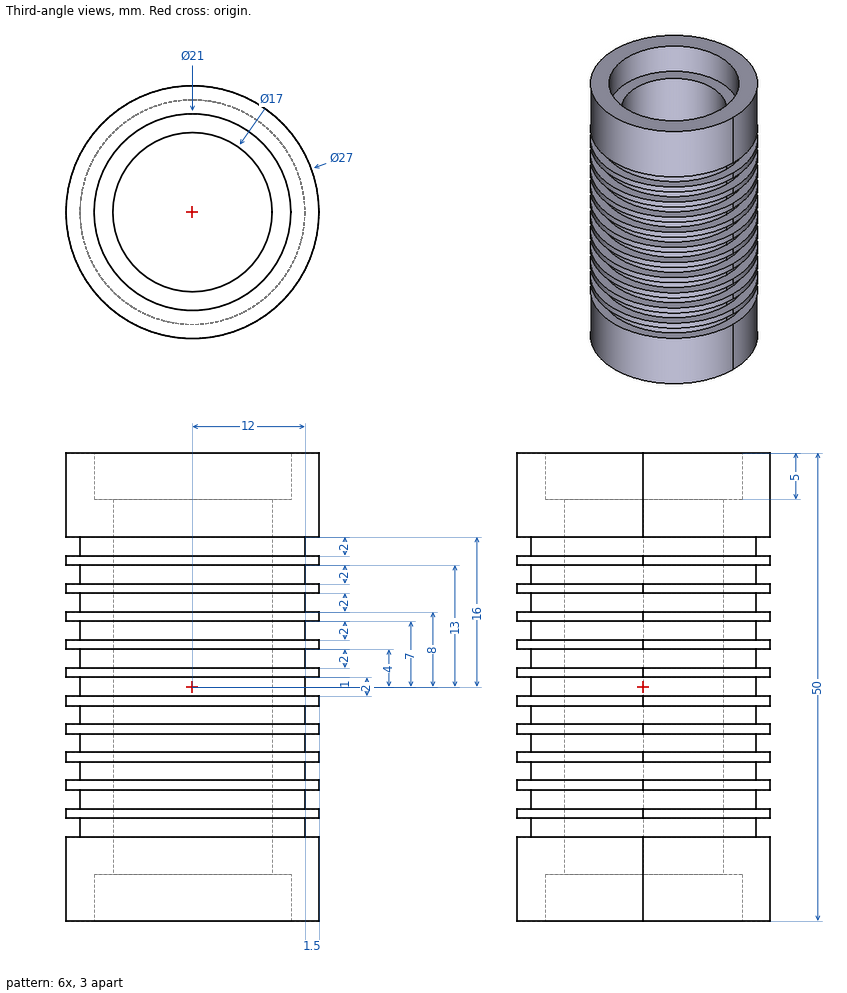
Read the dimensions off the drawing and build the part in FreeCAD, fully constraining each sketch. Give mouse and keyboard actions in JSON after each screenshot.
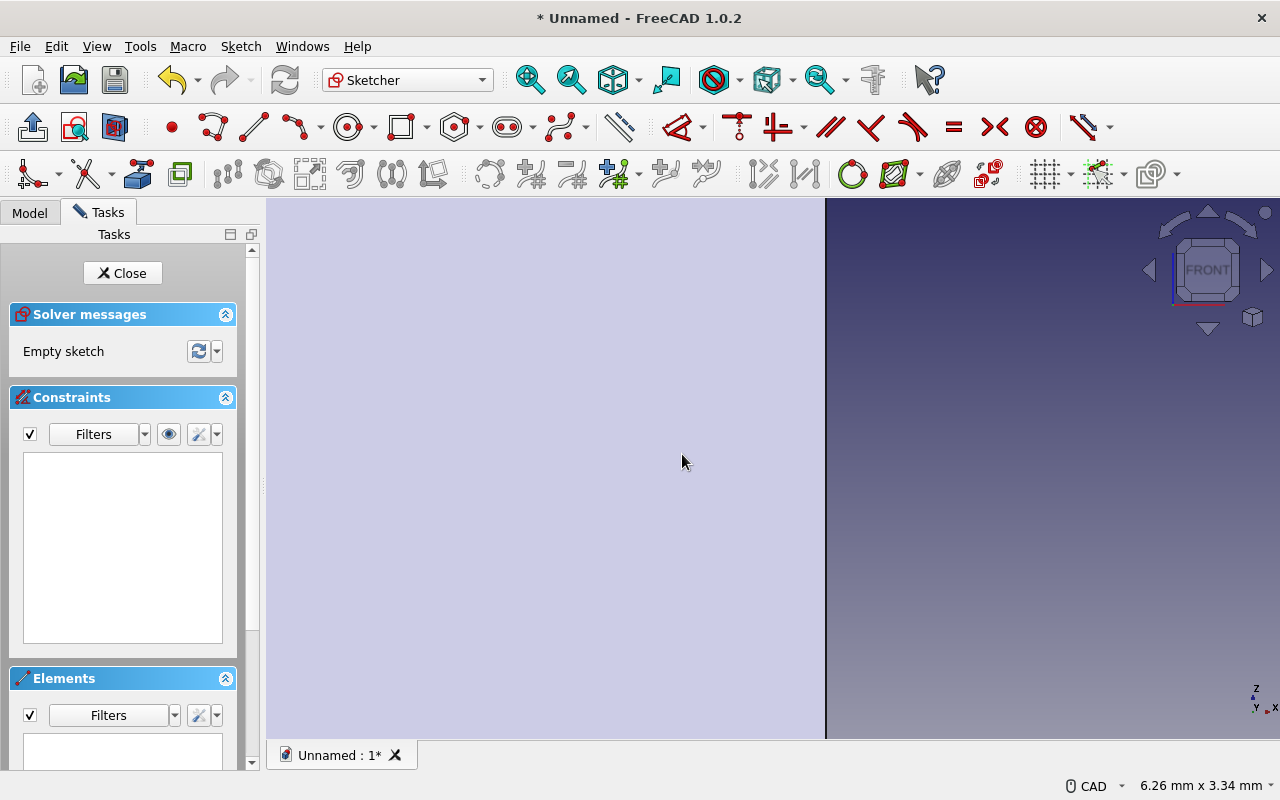
{"action": "left_click", "coordinate": [400, 128]}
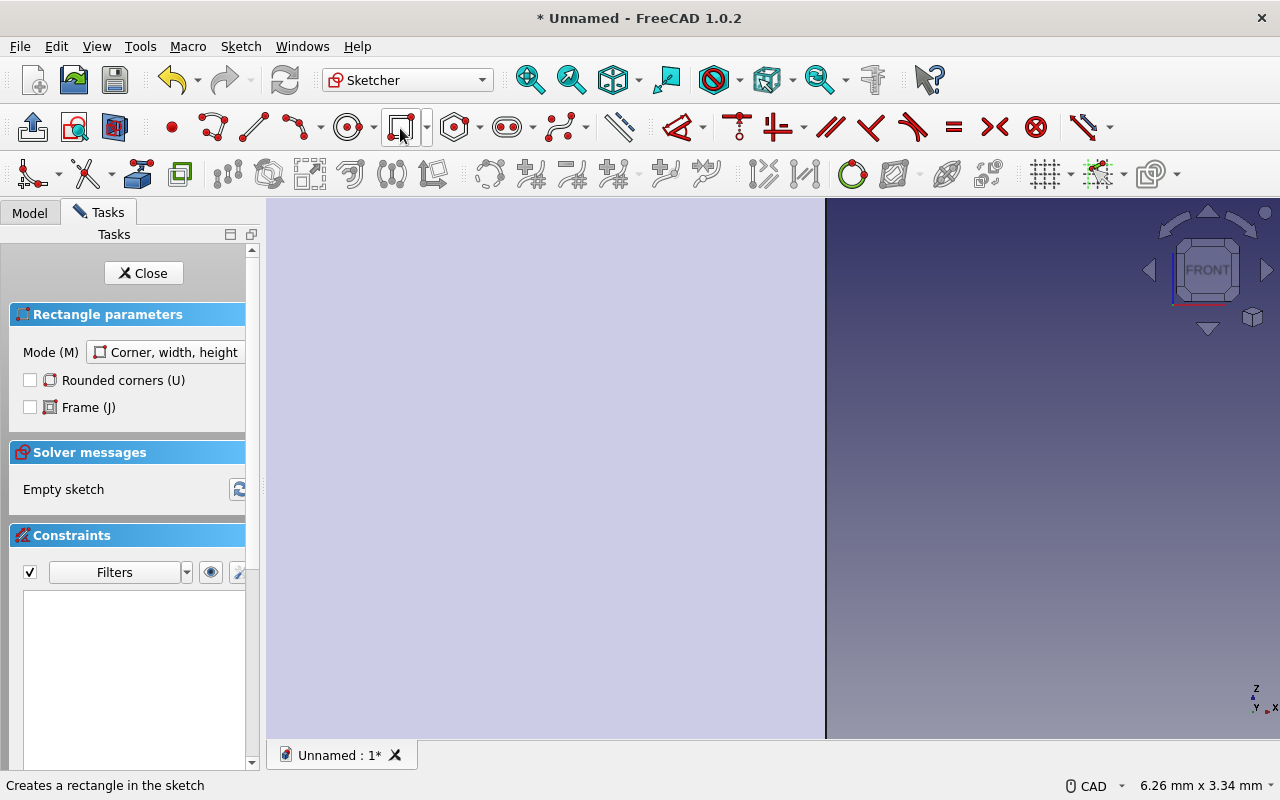
{"action": "left_click", "coordinate": [583, 306]}
{"action": "mouse_move", "coordinate": [826, 631]}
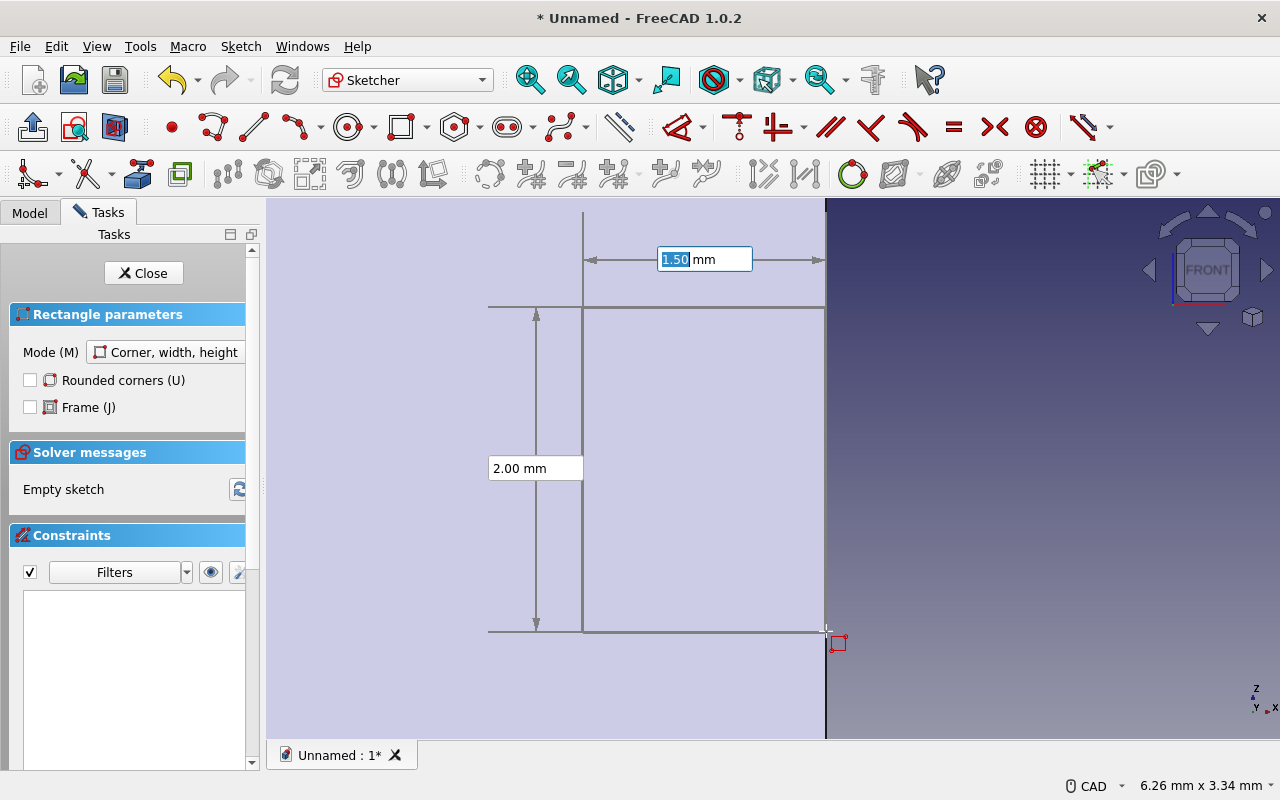
{"action": "type", "text": "1.5"}
{"action": "key", "text": "Tab"}
{"action": "type", "text": "2"}
{"action": "key", "text": "Return"}
{"action": "key", "text": "Escape"}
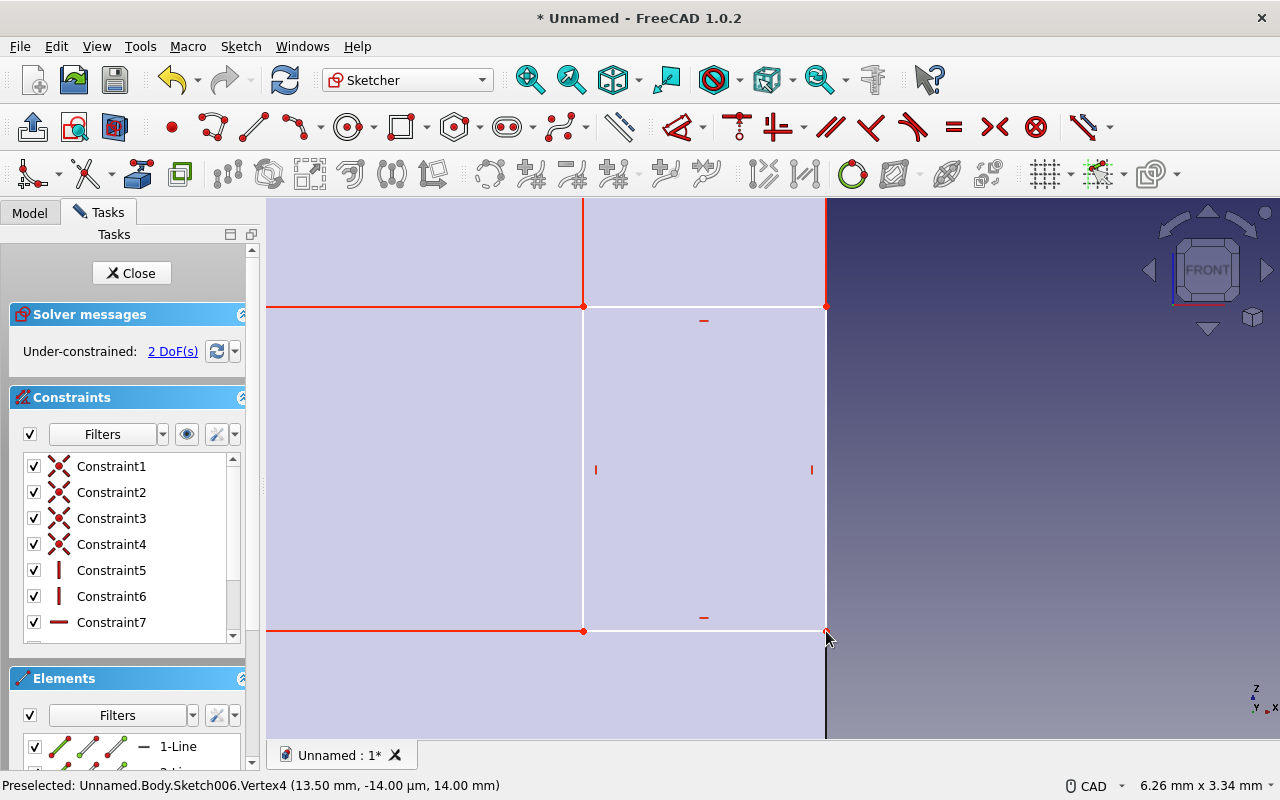
{"action": "key", "text": "d"}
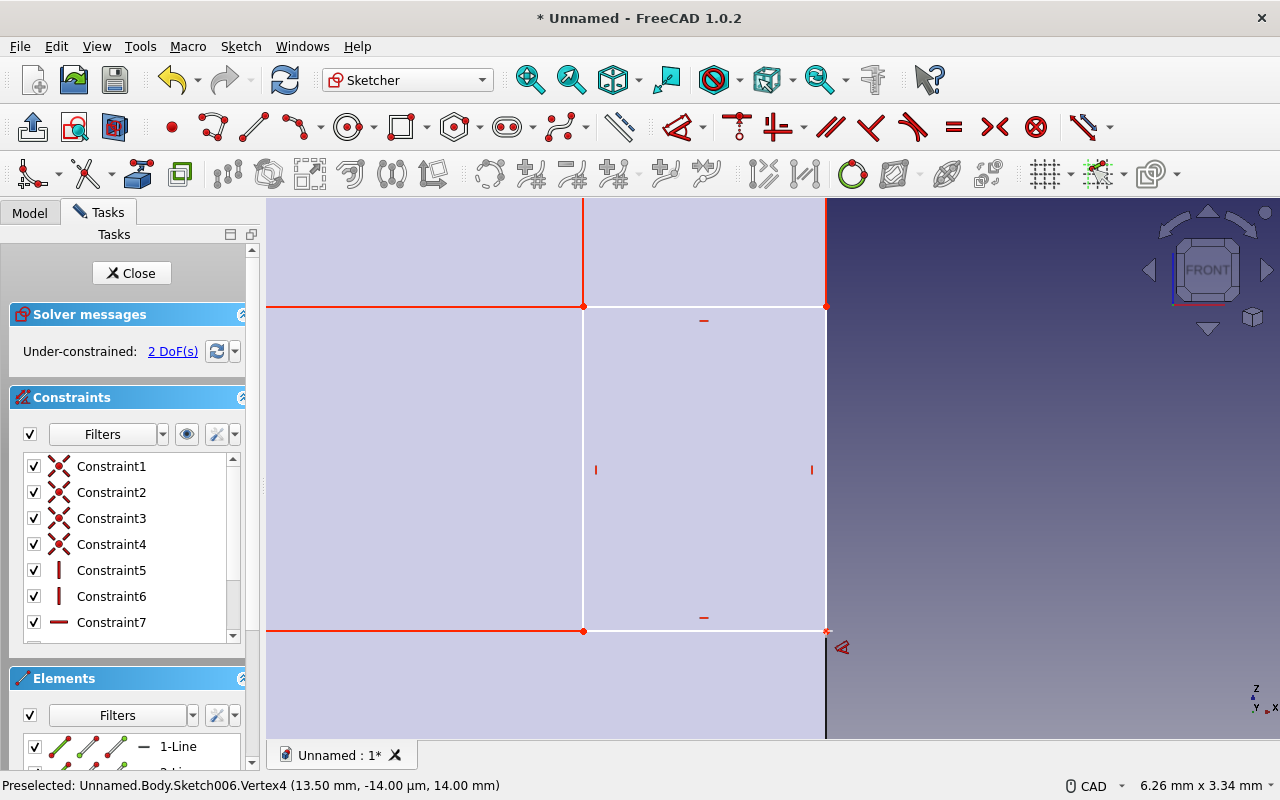
{"action": "left_click", "coordinate": [583, 307]}
{"action": "left_click", "coordinate": [438, 273]}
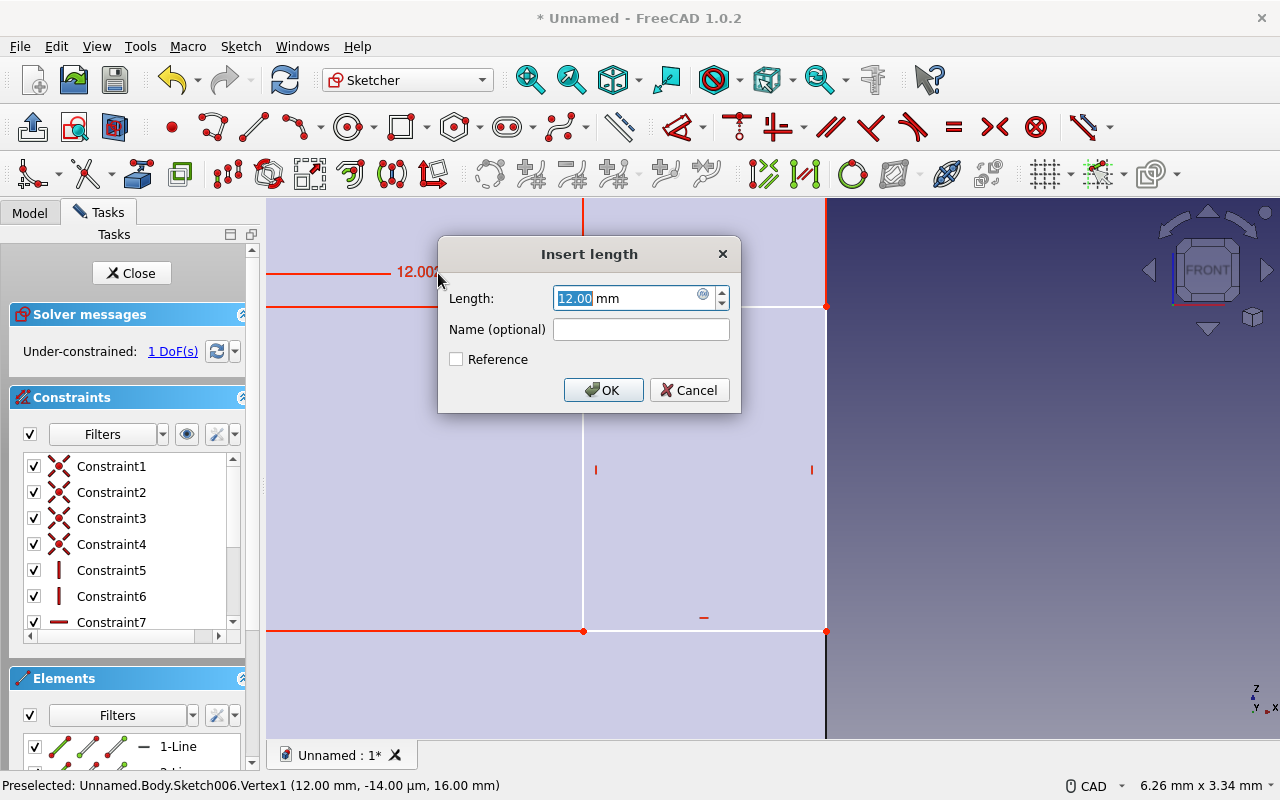
{"action": "type", "text": "12"}
{"action": "key", "text": "Return"}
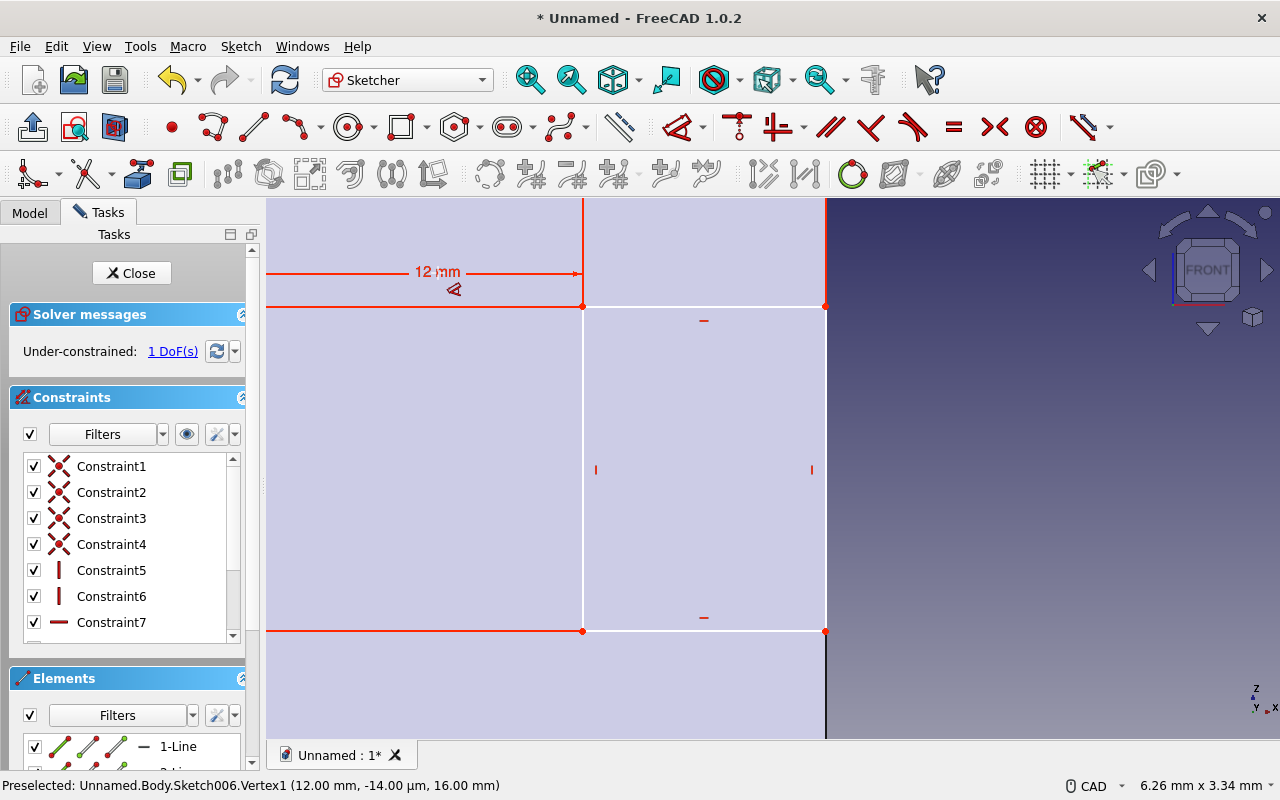
{"action": "left_click", "coordinate": [583, 307]}
{"action": "left_click", "coordinate": [617, 509]}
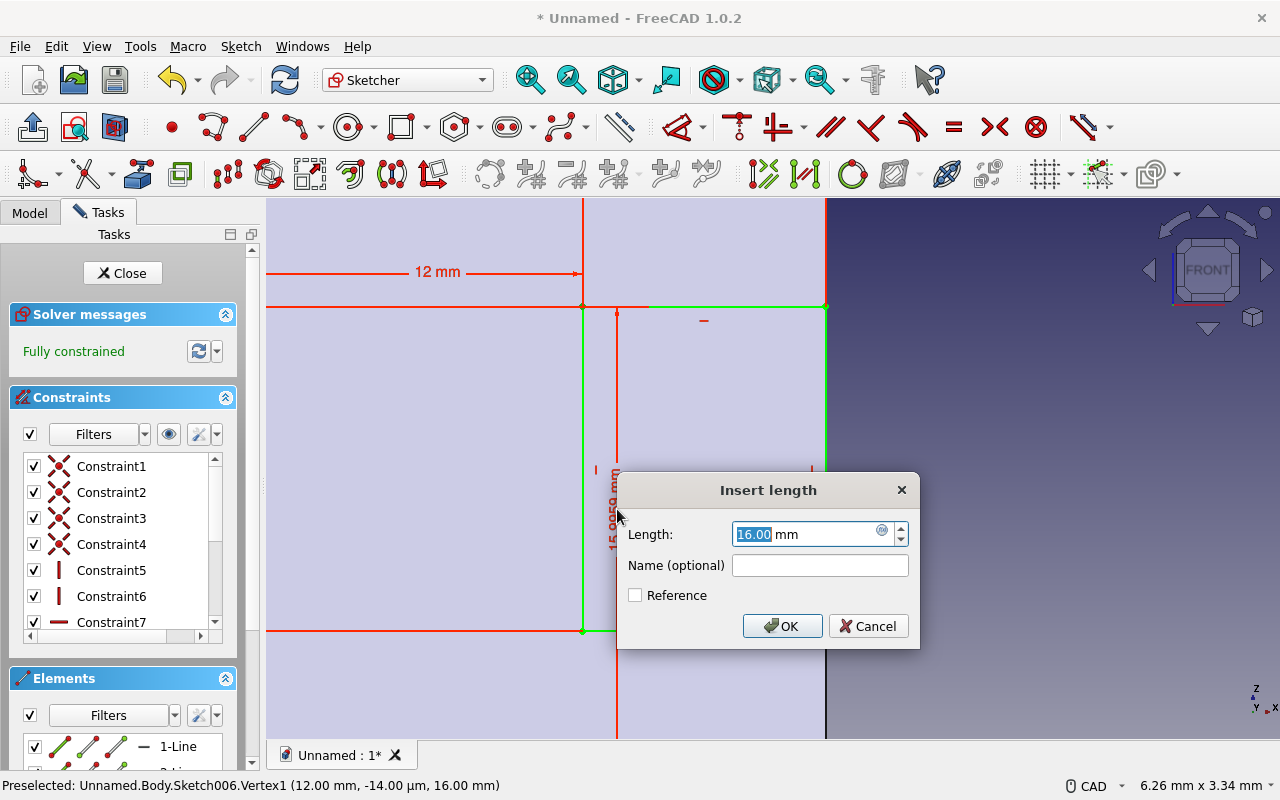
{"action": "type", "text": "16"}
{"action": "key", "text": "Return"}
{"action": "key", "text": "Escape"}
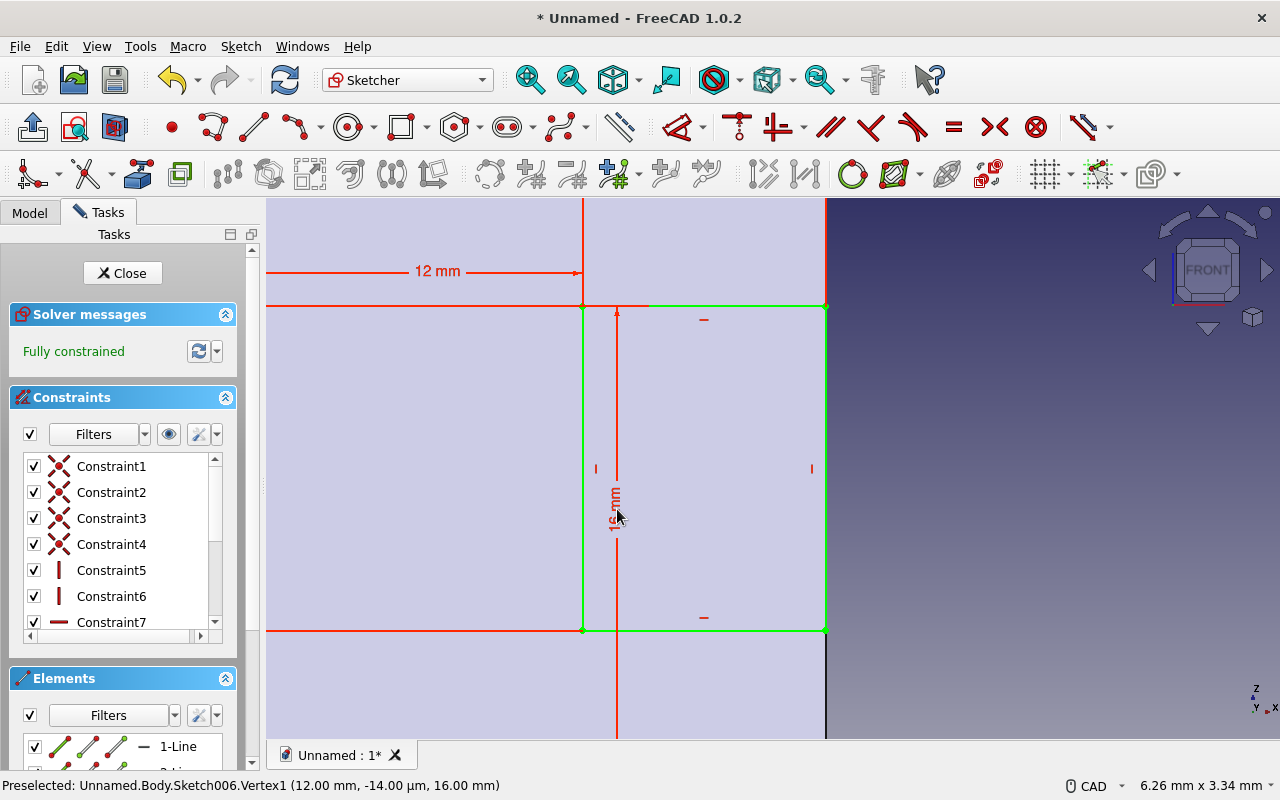
{"action": "left_click", "coordinate": [123, 273]}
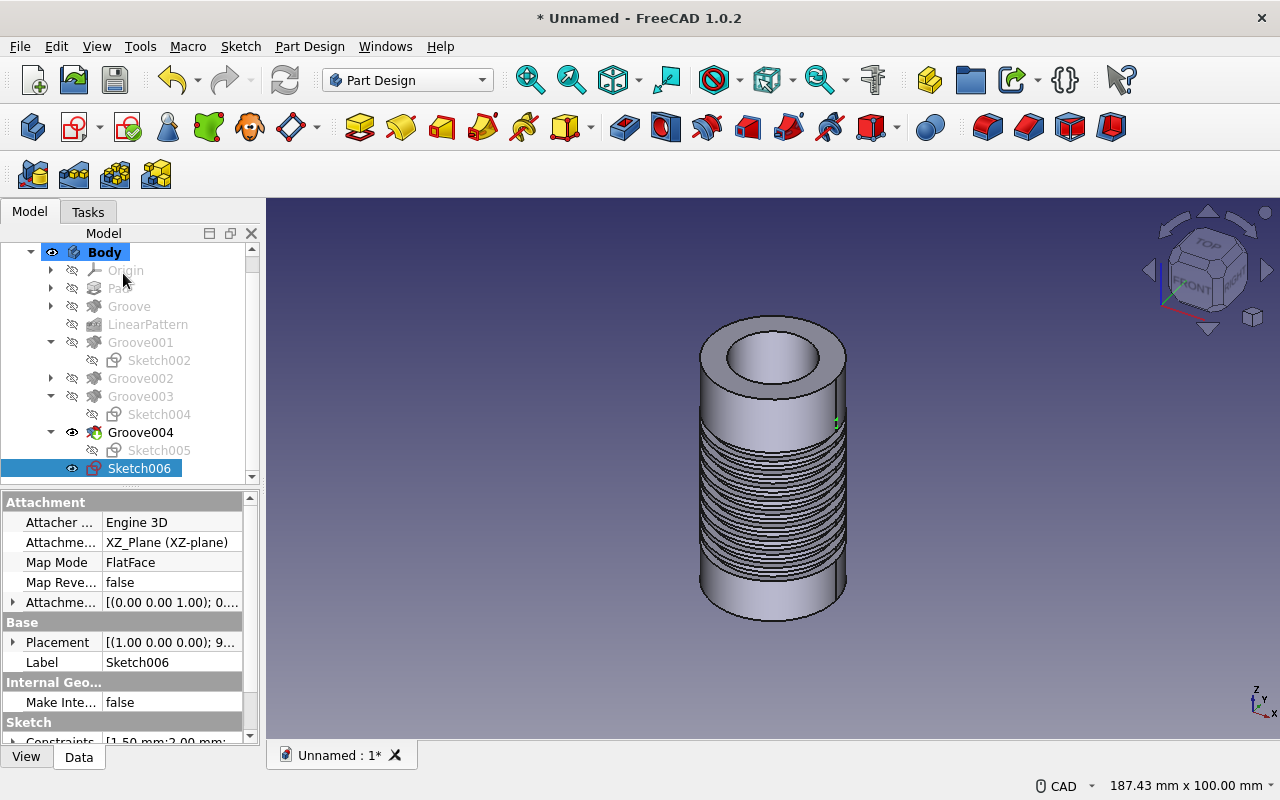
{"action": "left_click", "coordinate": [707, 128]}